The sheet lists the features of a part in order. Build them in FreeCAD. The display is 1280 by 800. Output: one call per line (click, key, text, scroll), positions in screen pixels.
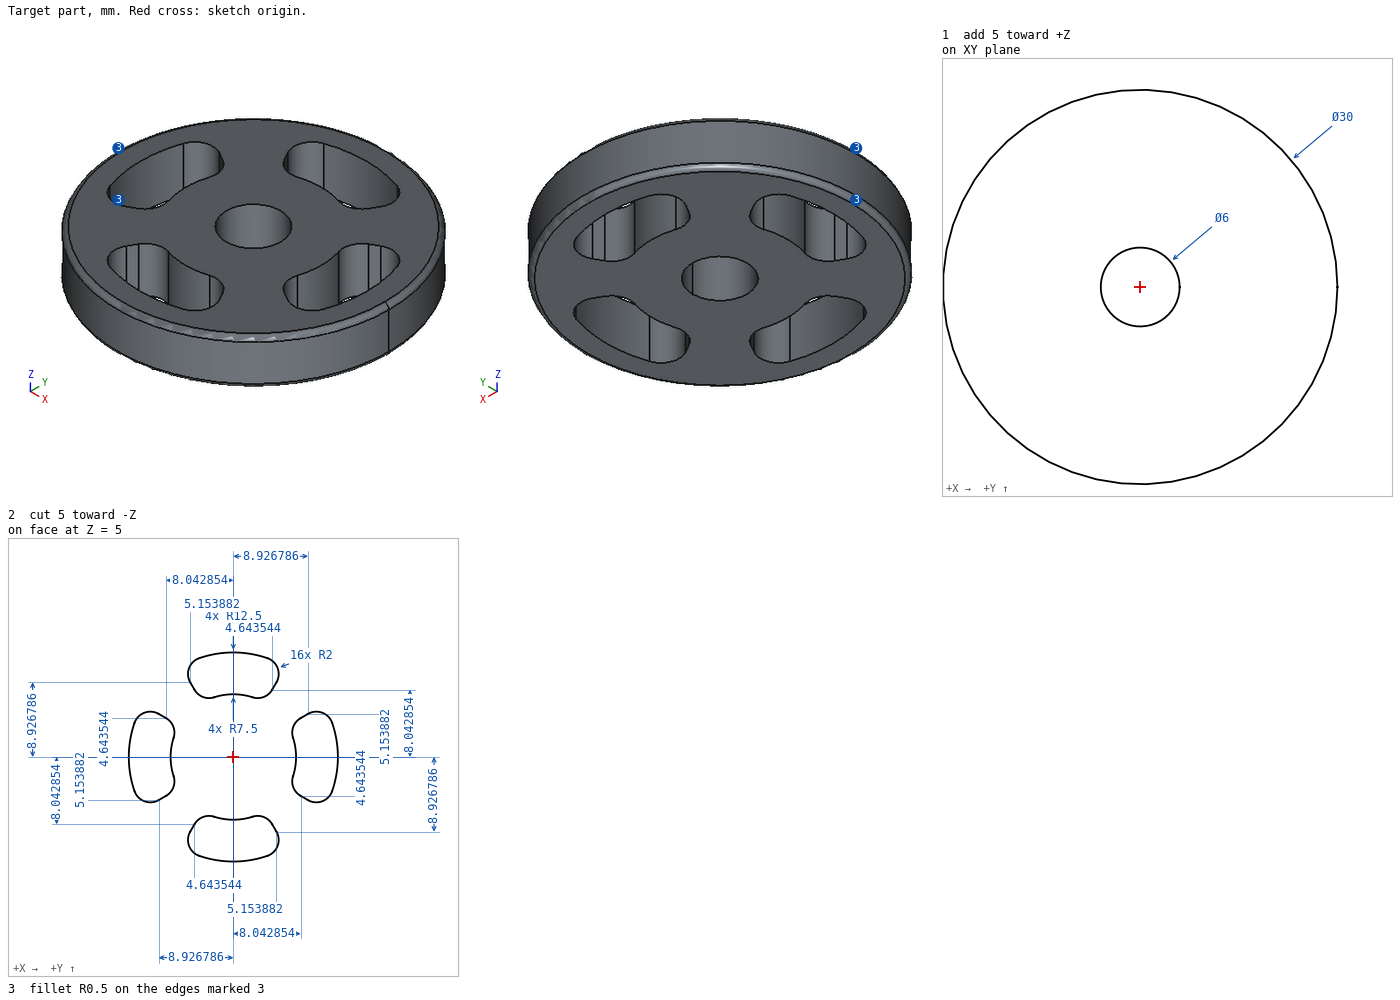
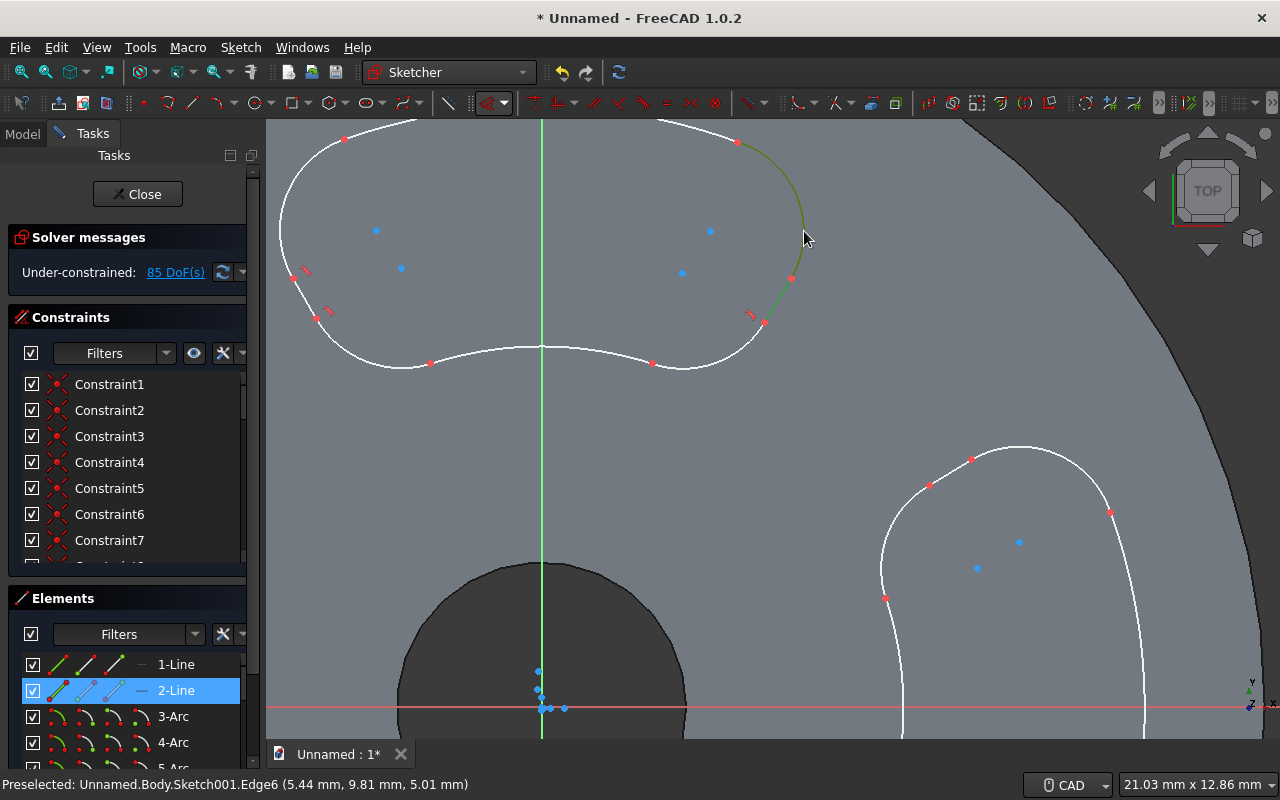
click(644, 104)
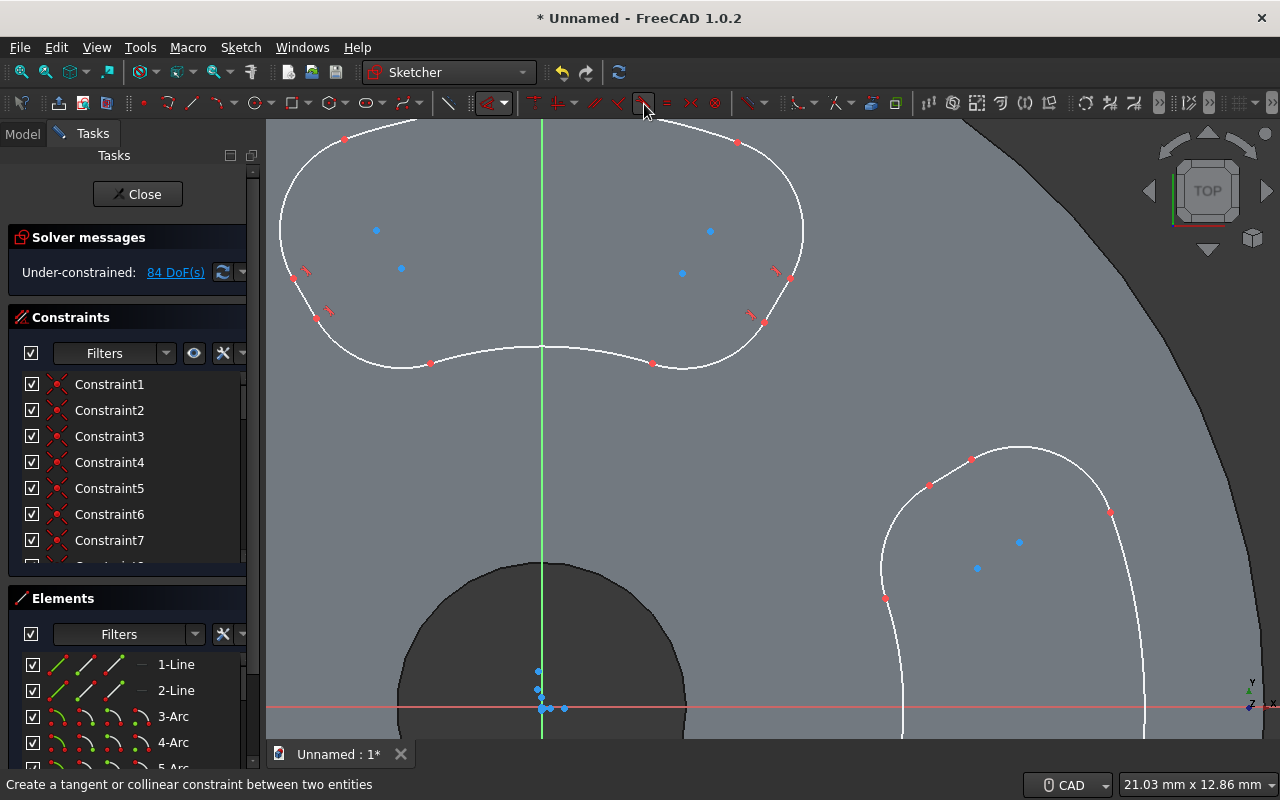
click(343, 348)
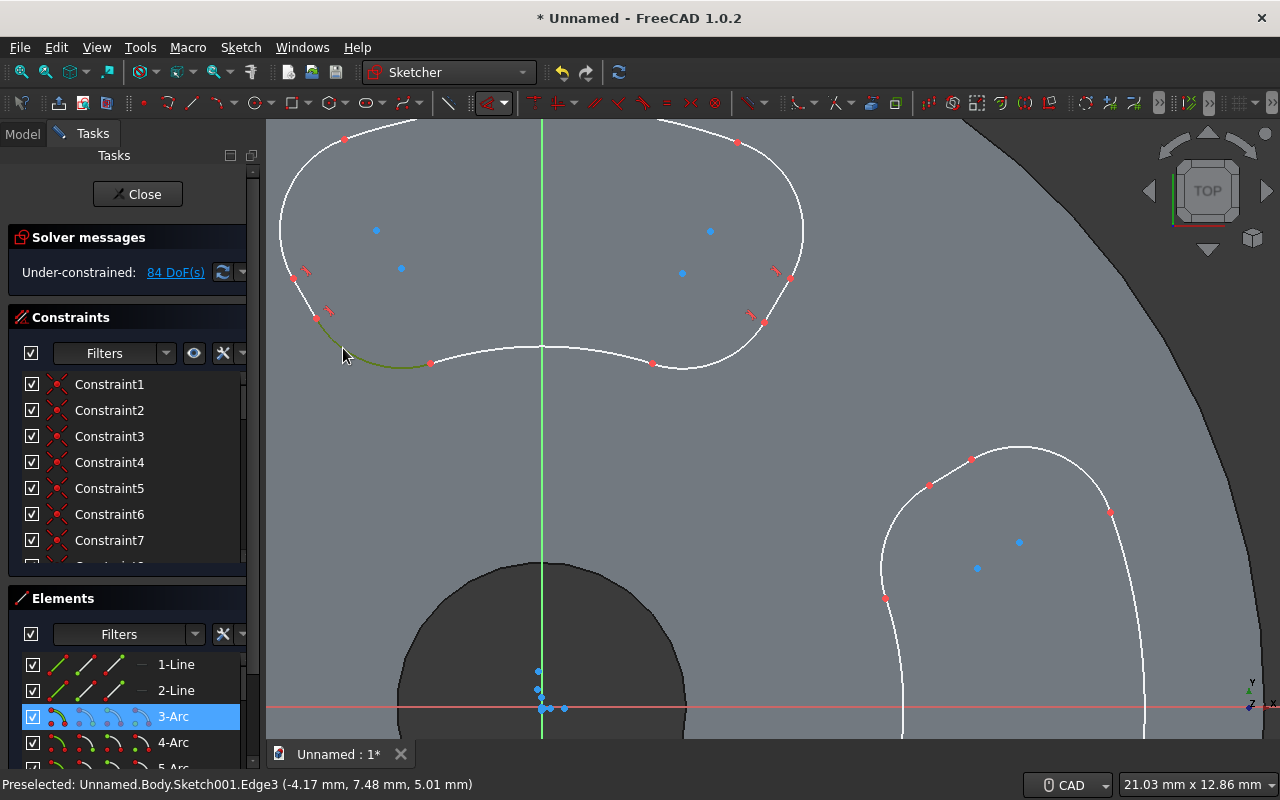
click(587, 349)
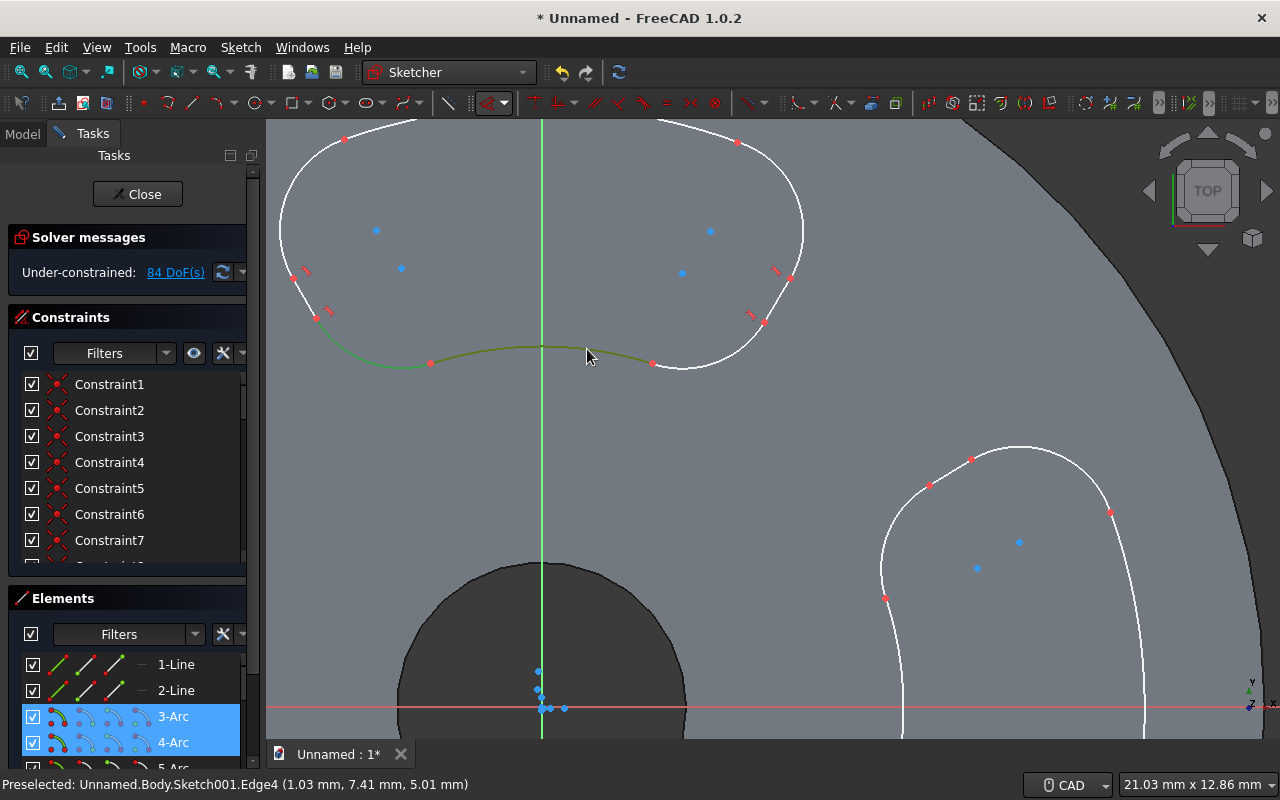
click(644, 104)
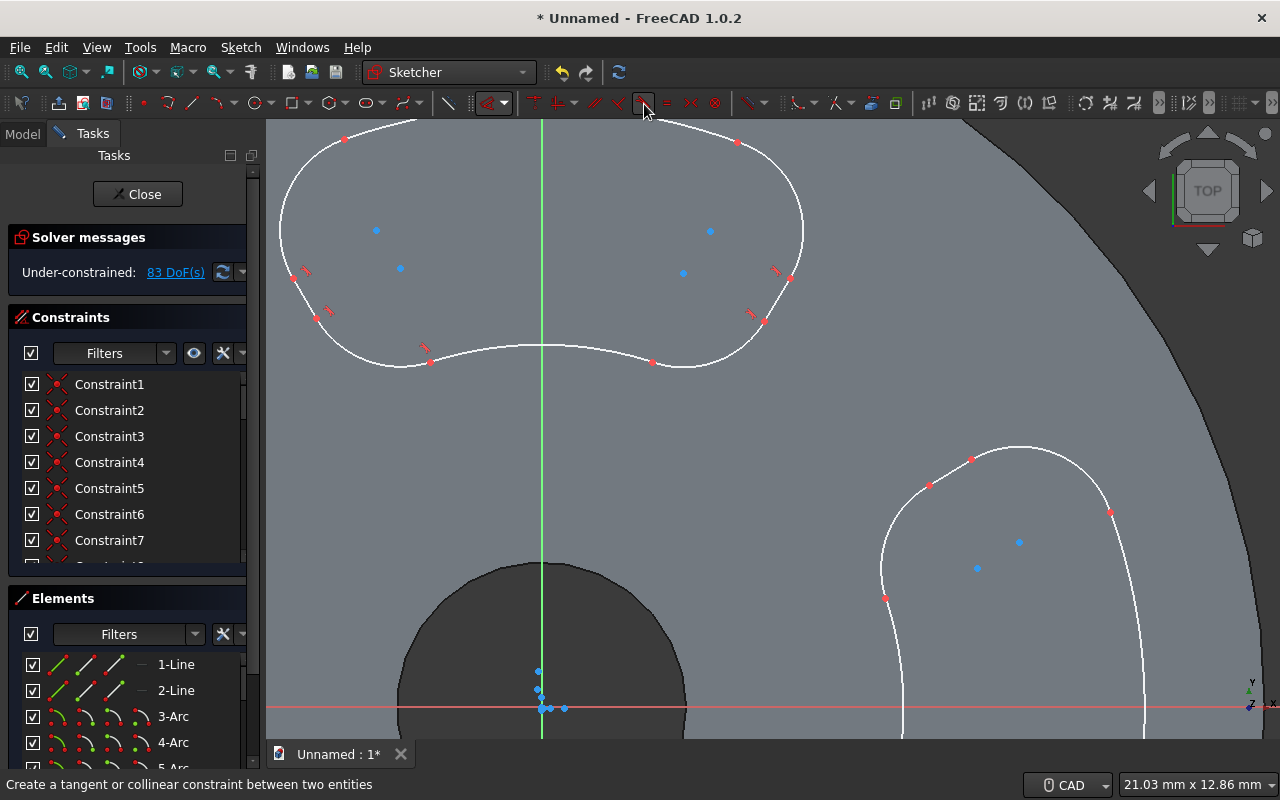
click(587, 348)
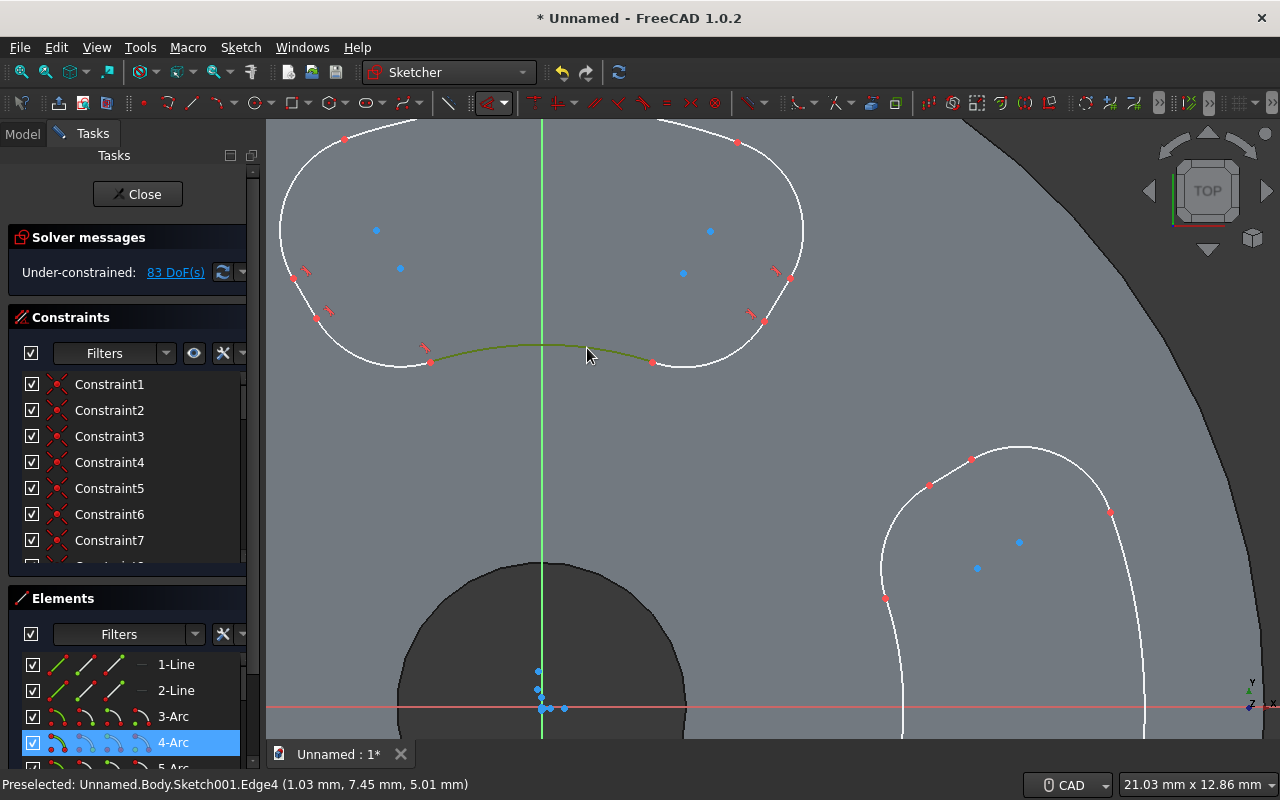
click(691, 367)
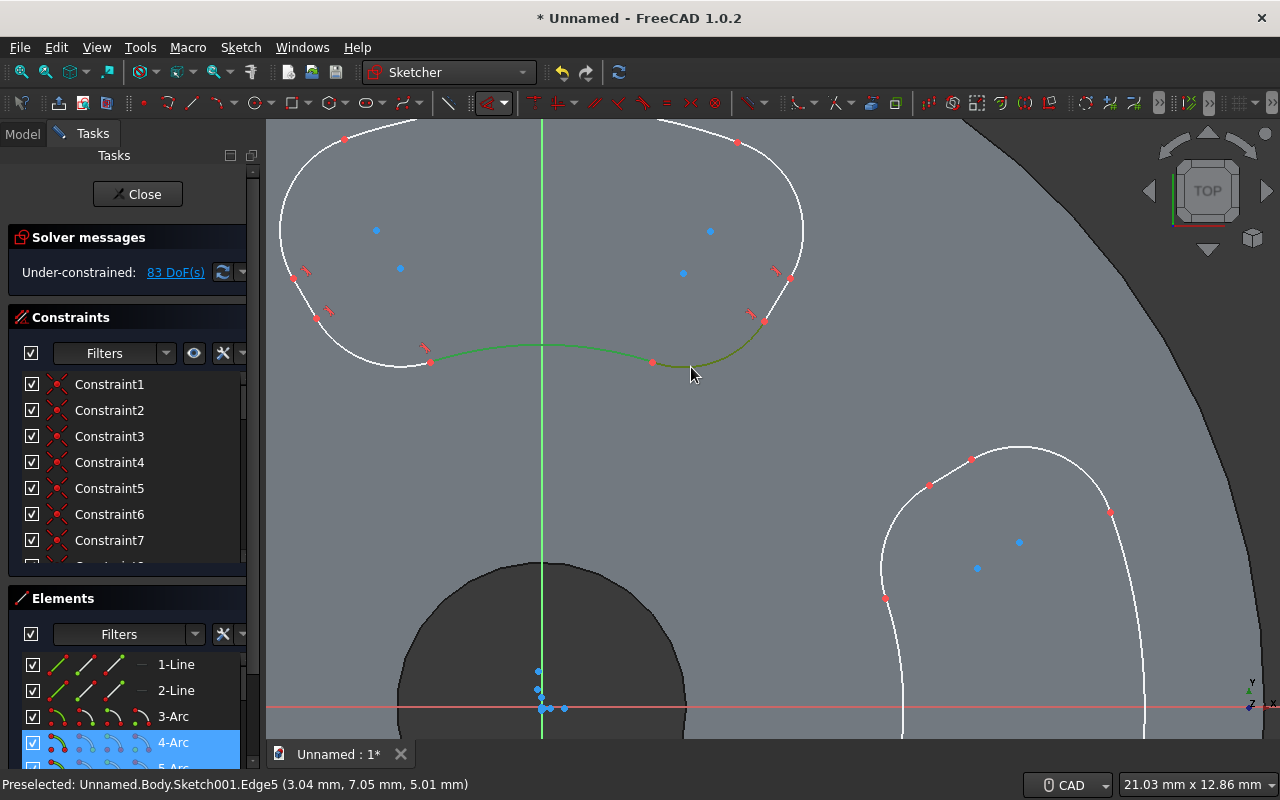
click(644, 104)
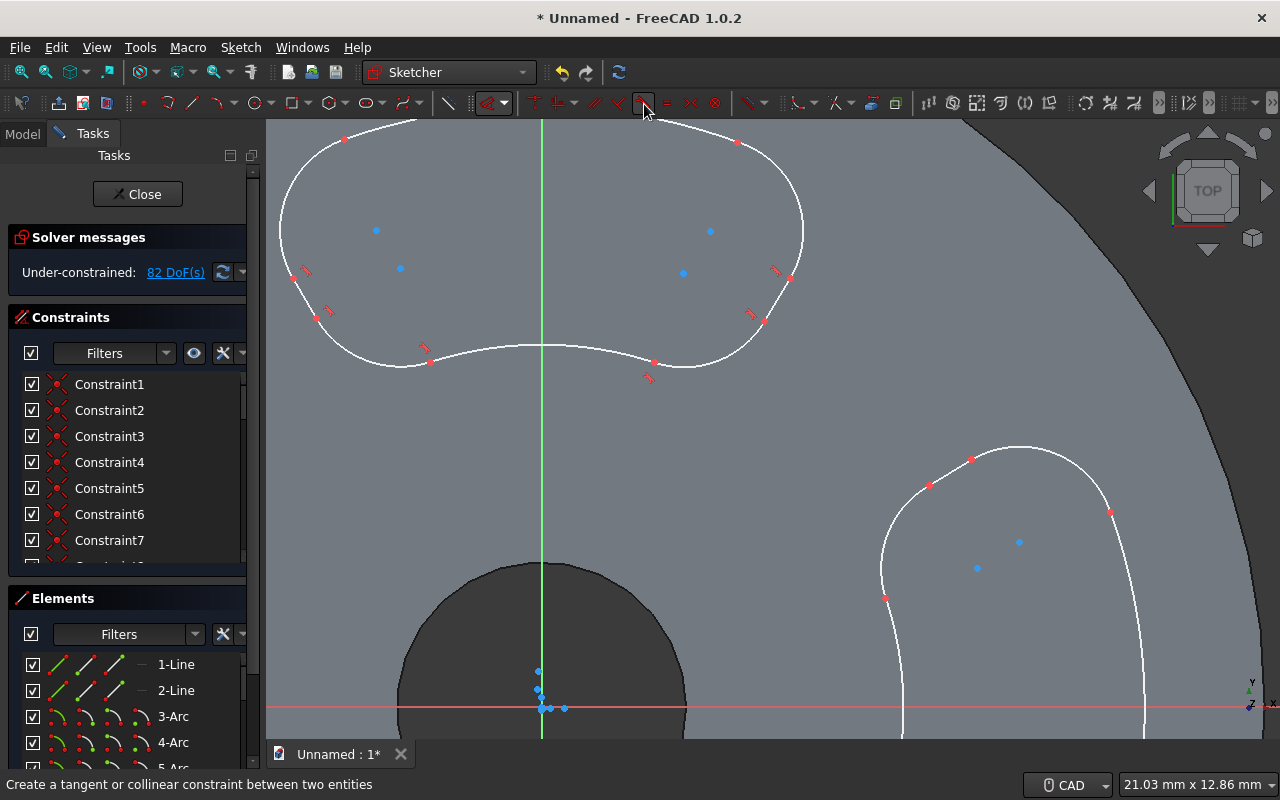
click(803, 231)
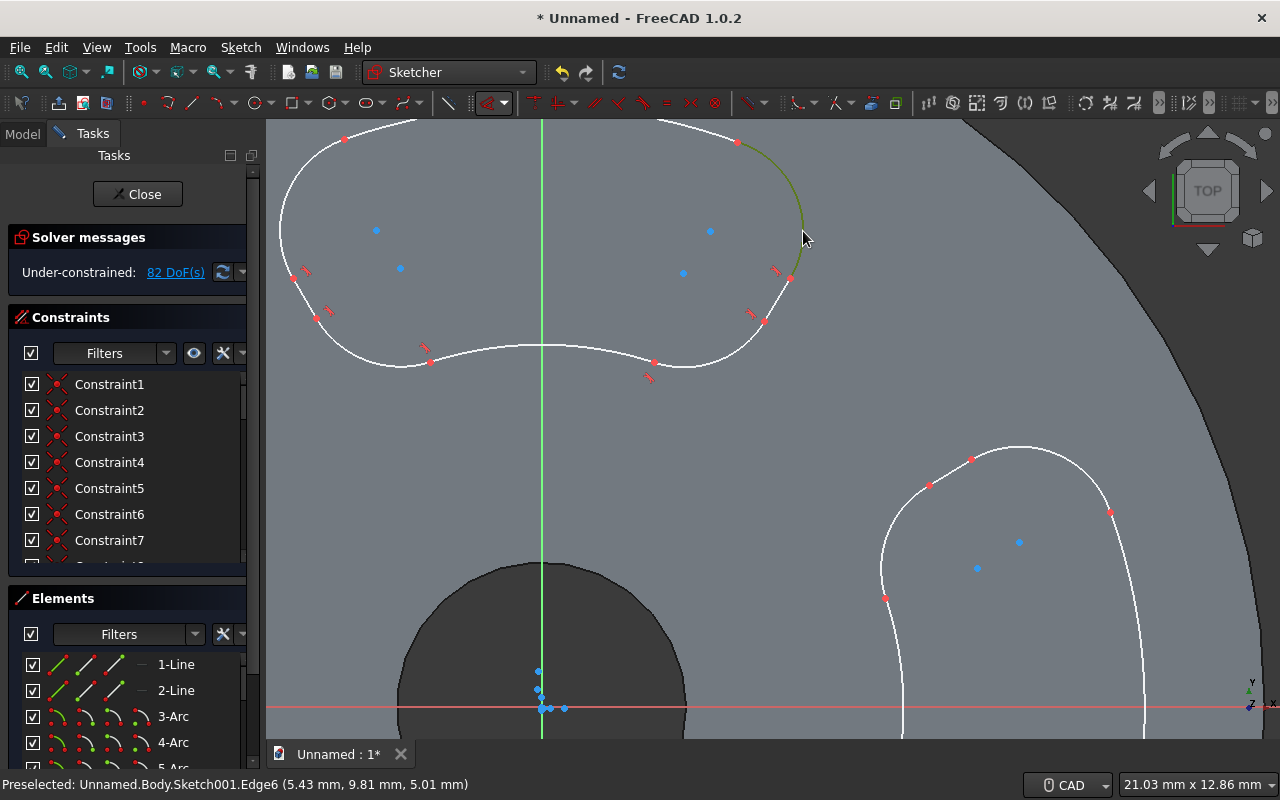
scroll(775, 309, down, 6)